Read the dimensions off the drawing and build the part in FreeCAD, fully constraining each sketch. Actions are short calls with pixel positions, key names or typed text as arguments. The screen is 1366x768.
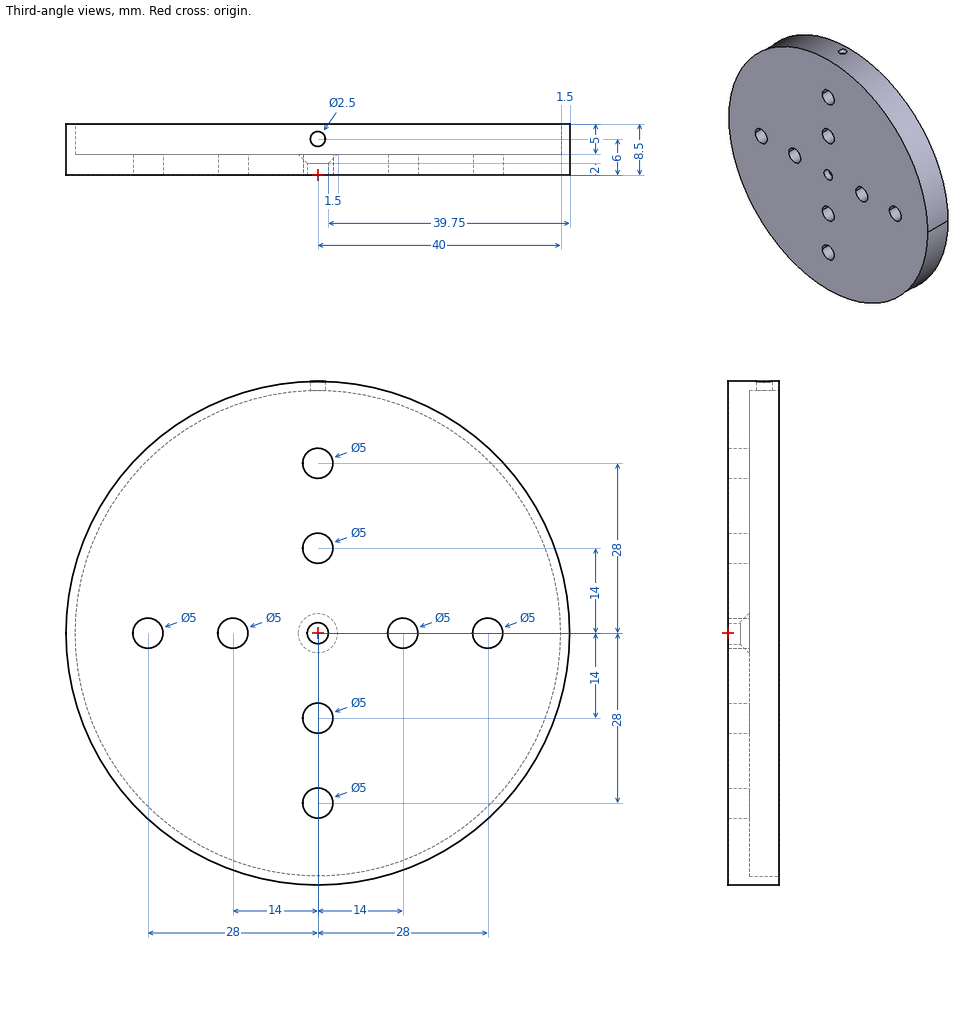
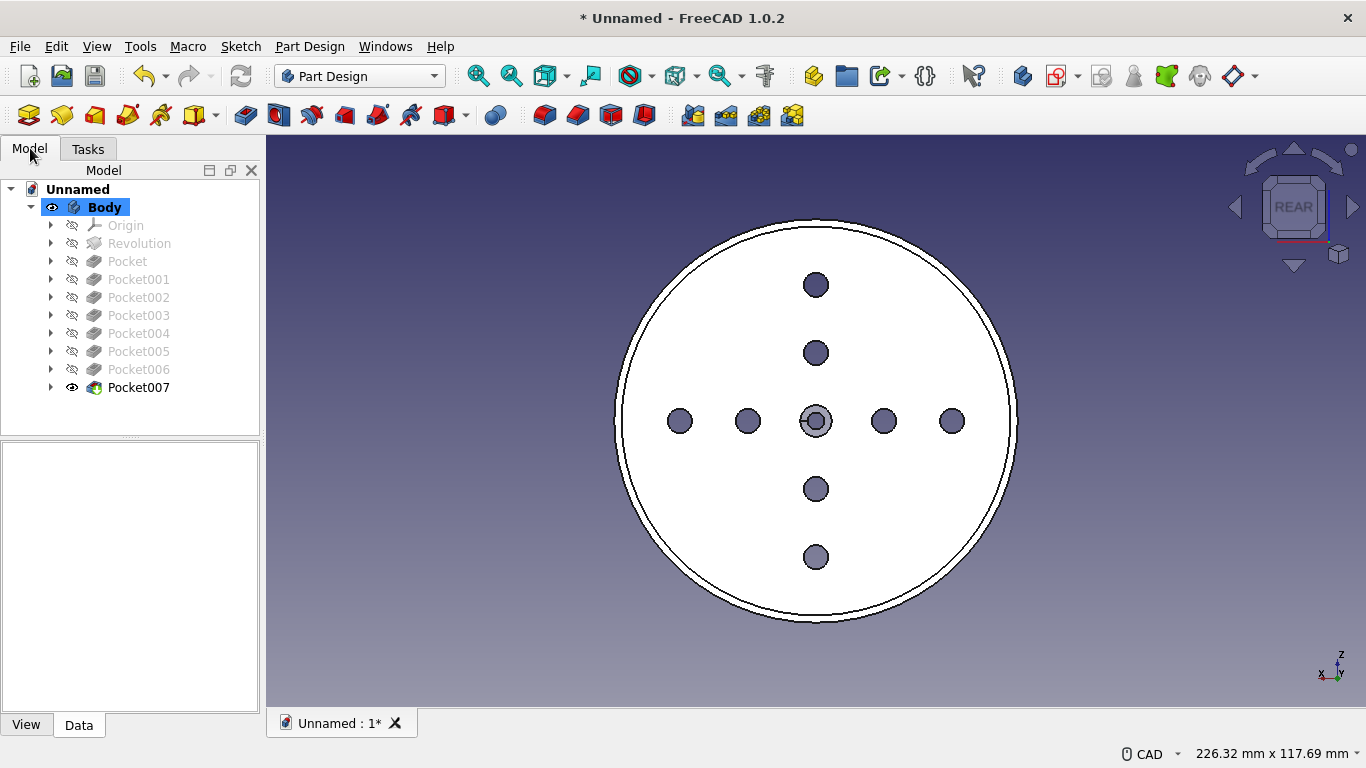
click(51, 225)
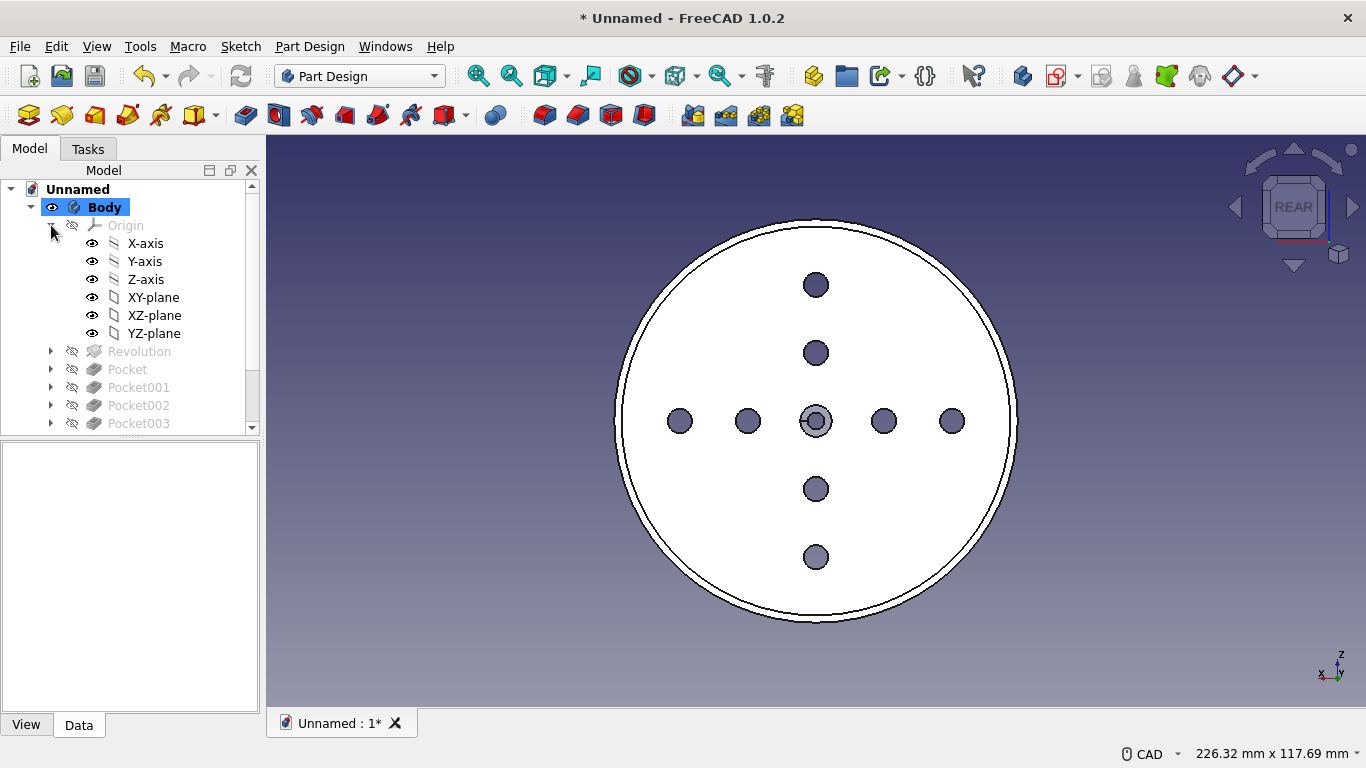
click(137, 297)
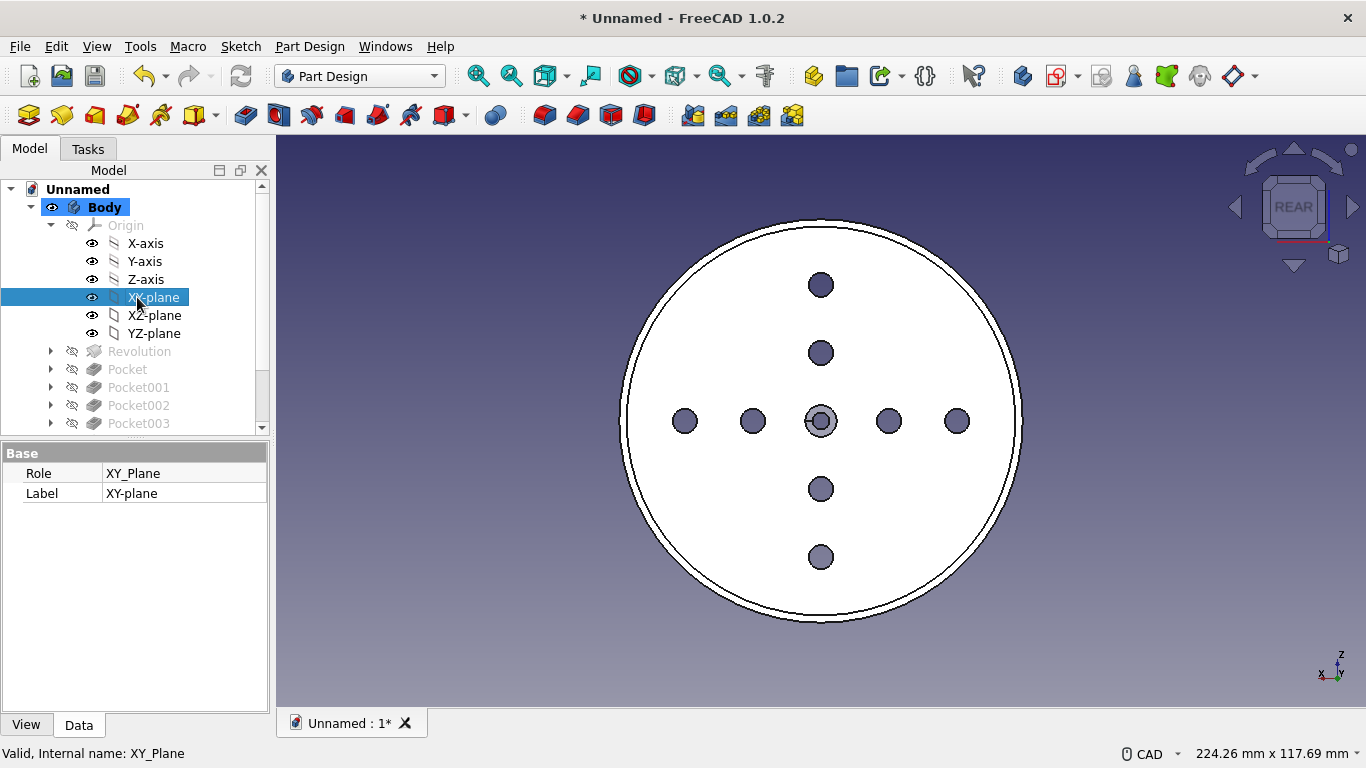
click(1232, 76)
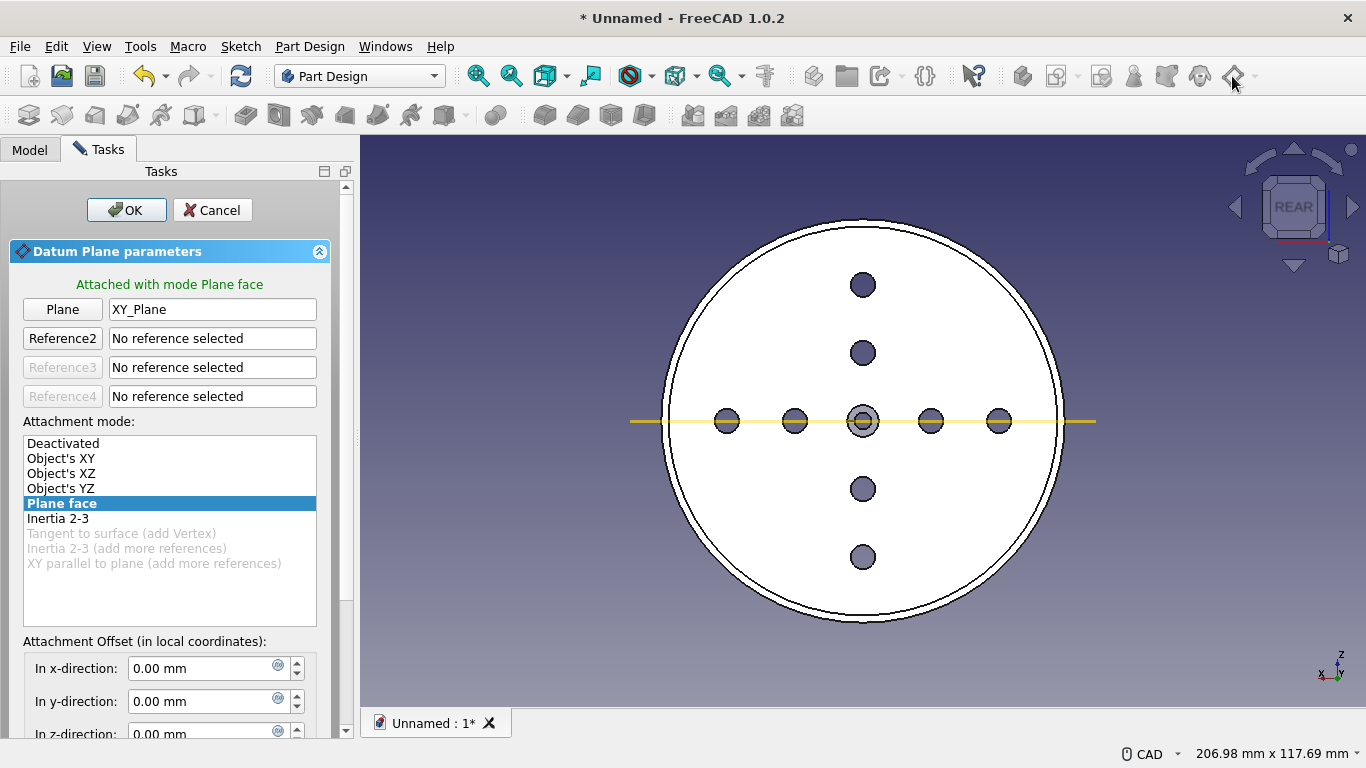
scroll(346, 460, down, 2)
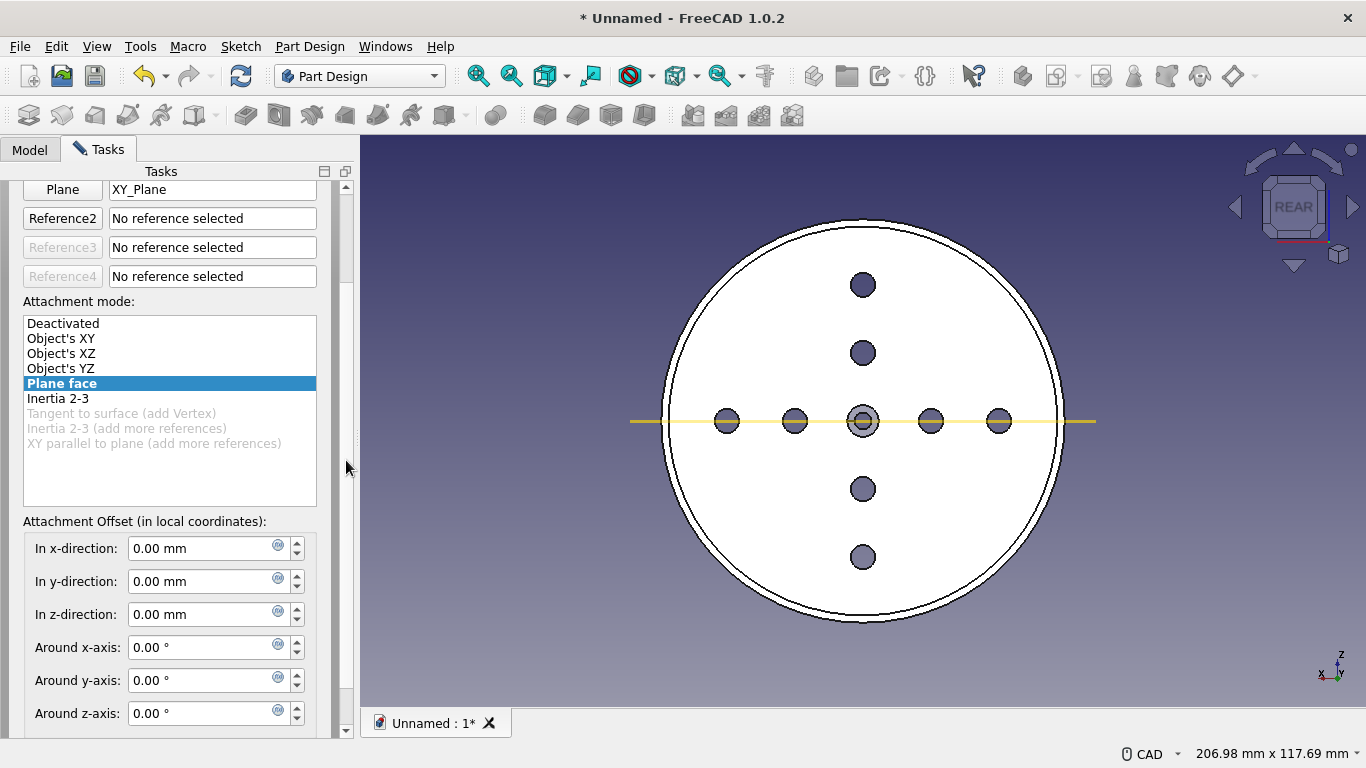
triple_click(210, 614)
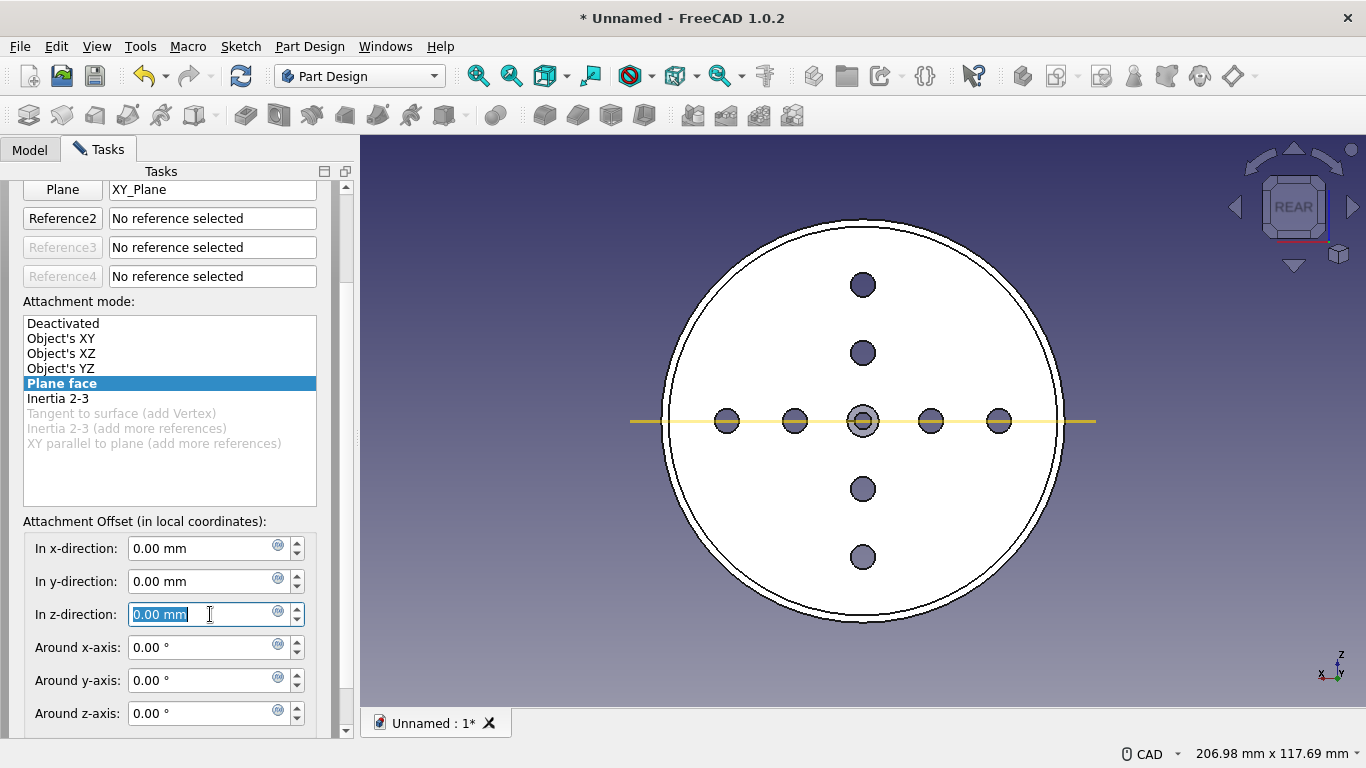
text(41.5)
key(Tab)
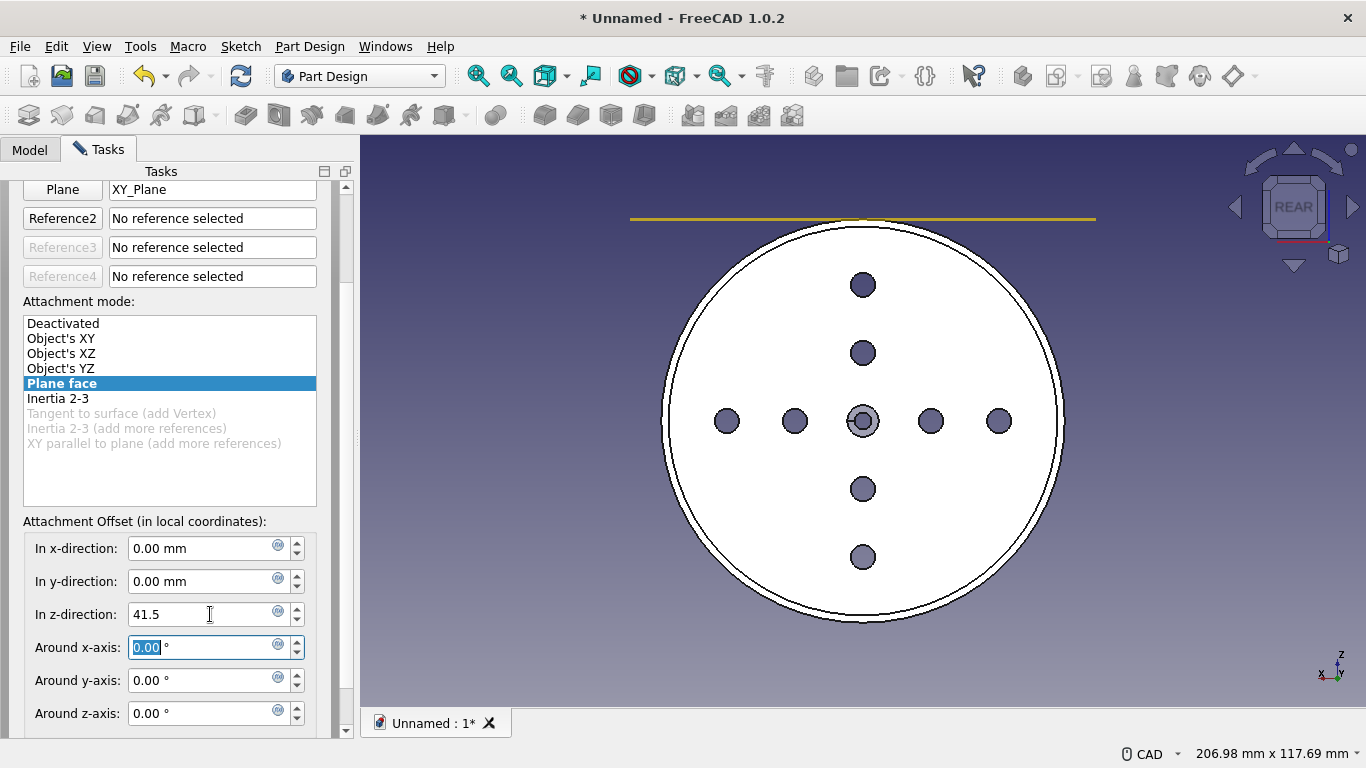
scroll(346, 460, up, 3)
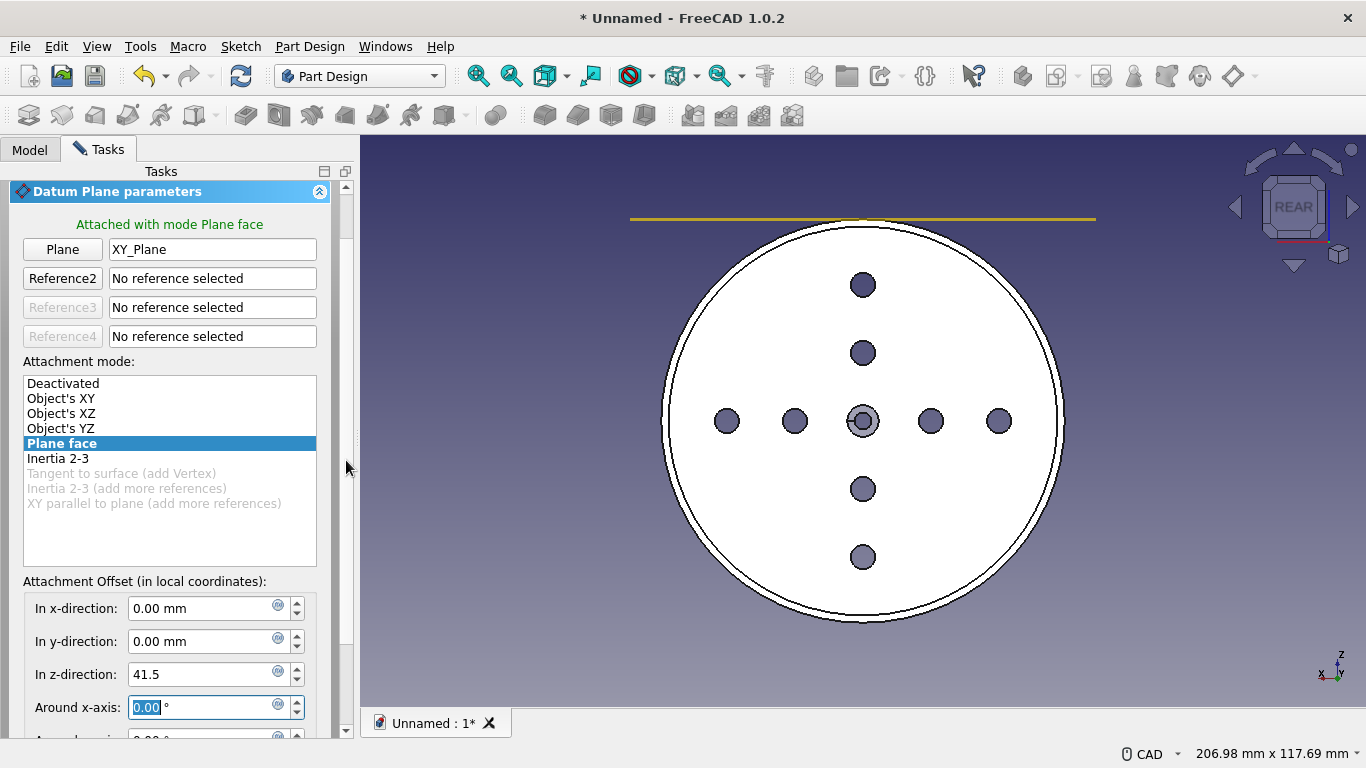
click(127, 210)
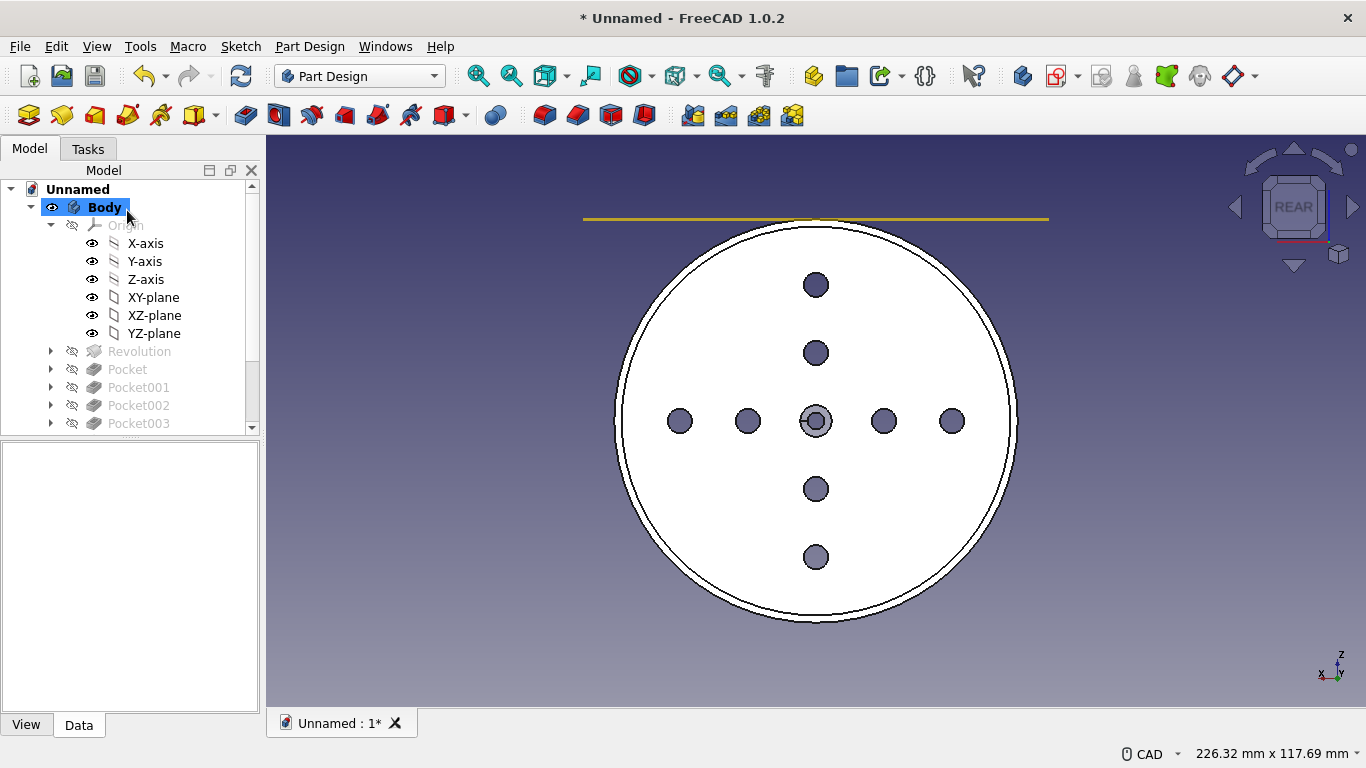
scroll(101, 311, down, 3)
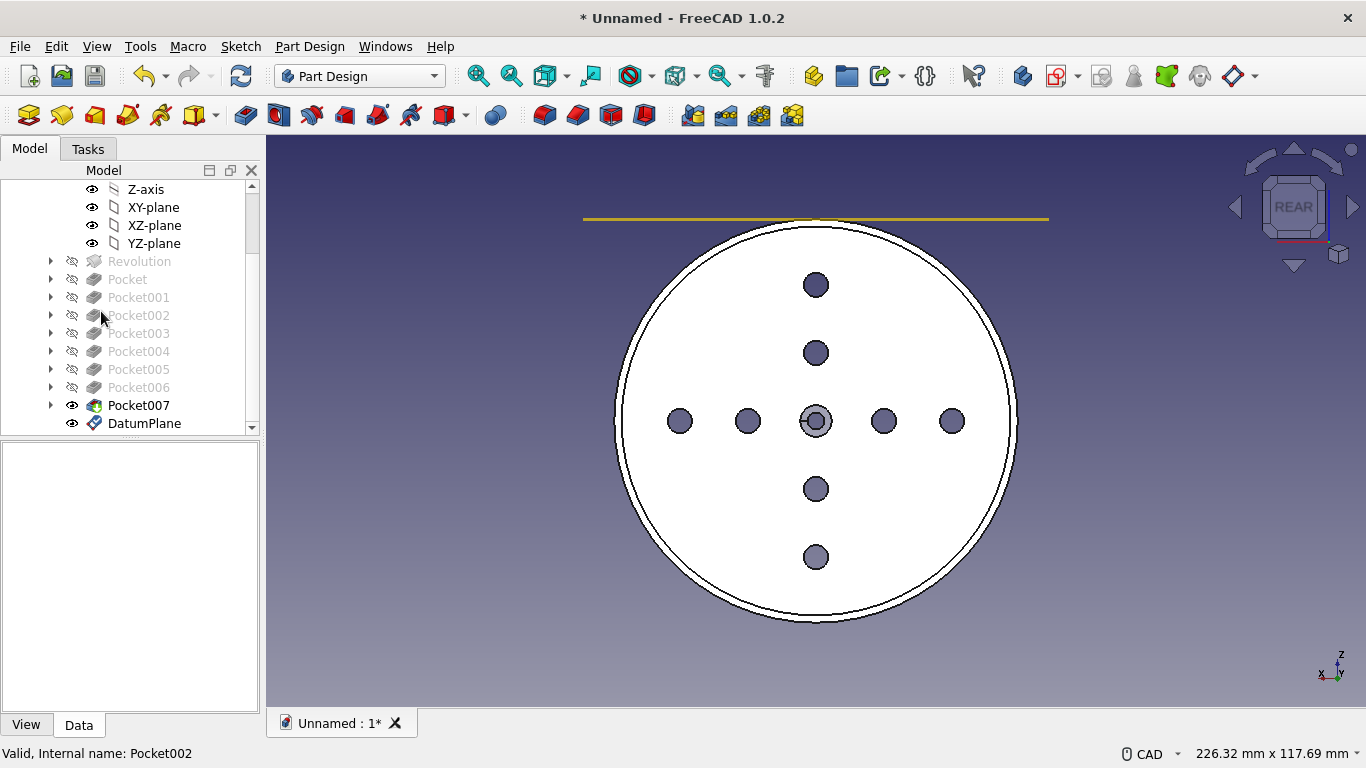
click(117, 423)